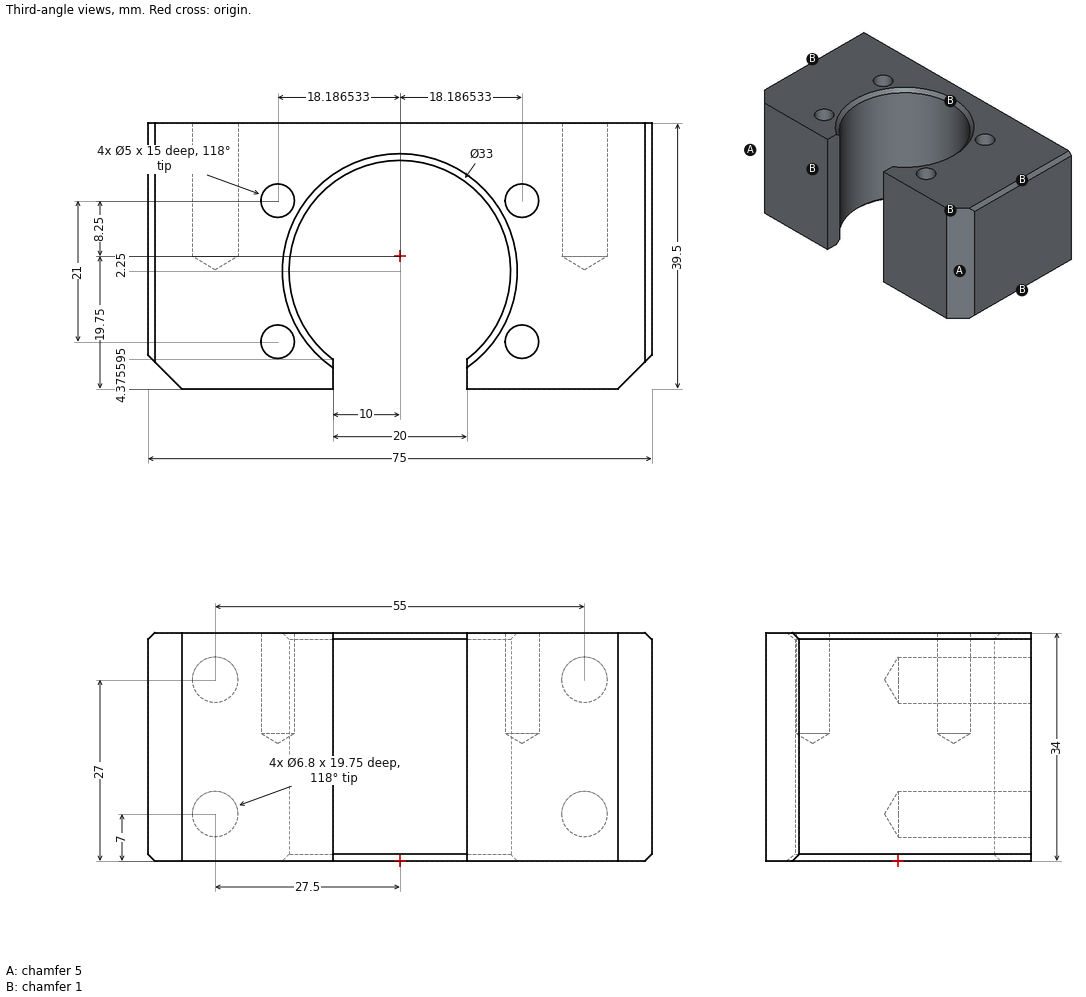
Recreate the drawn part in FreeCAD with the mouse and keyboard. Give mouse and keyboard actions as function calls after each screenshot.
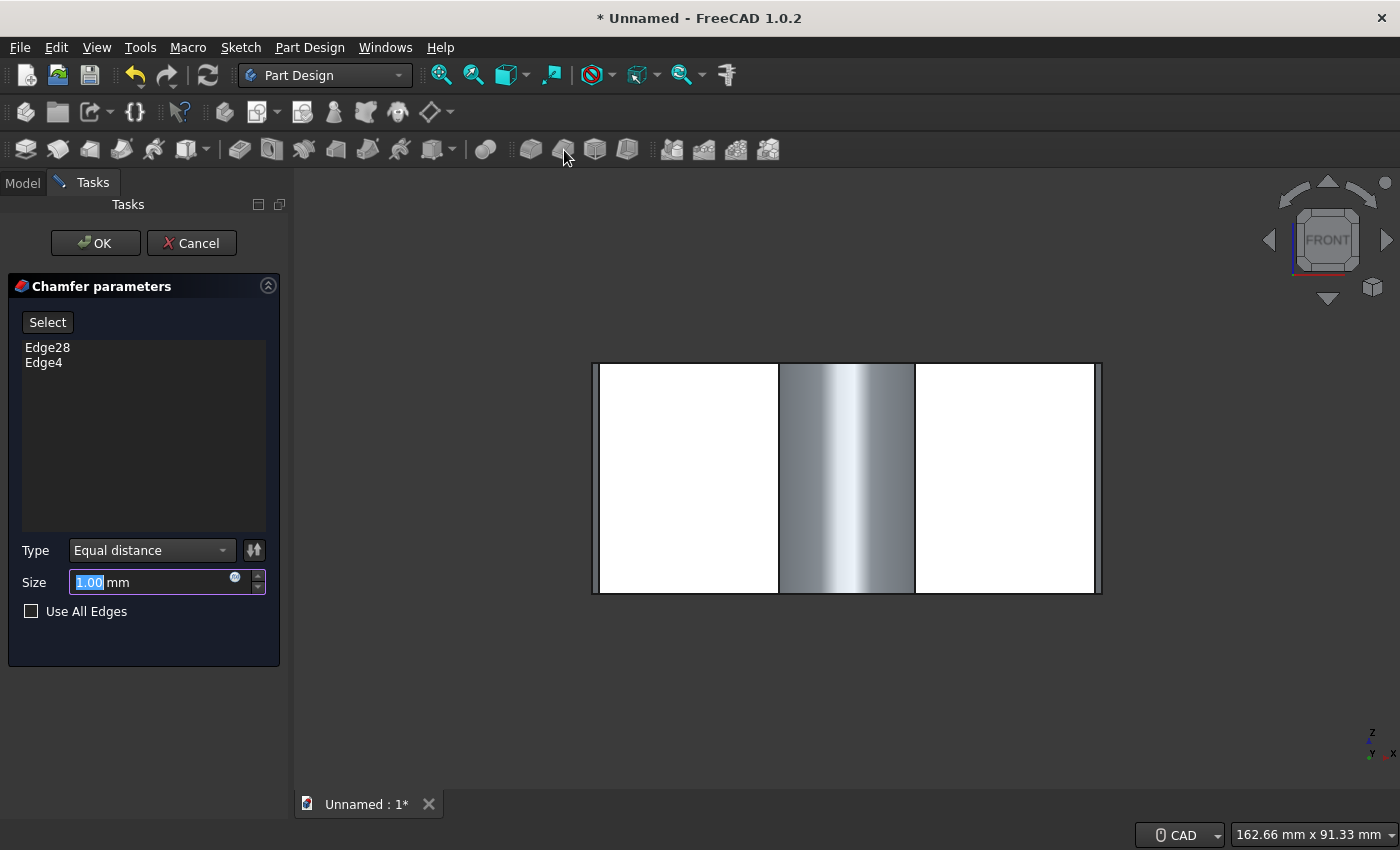
text(5)
key(Tab)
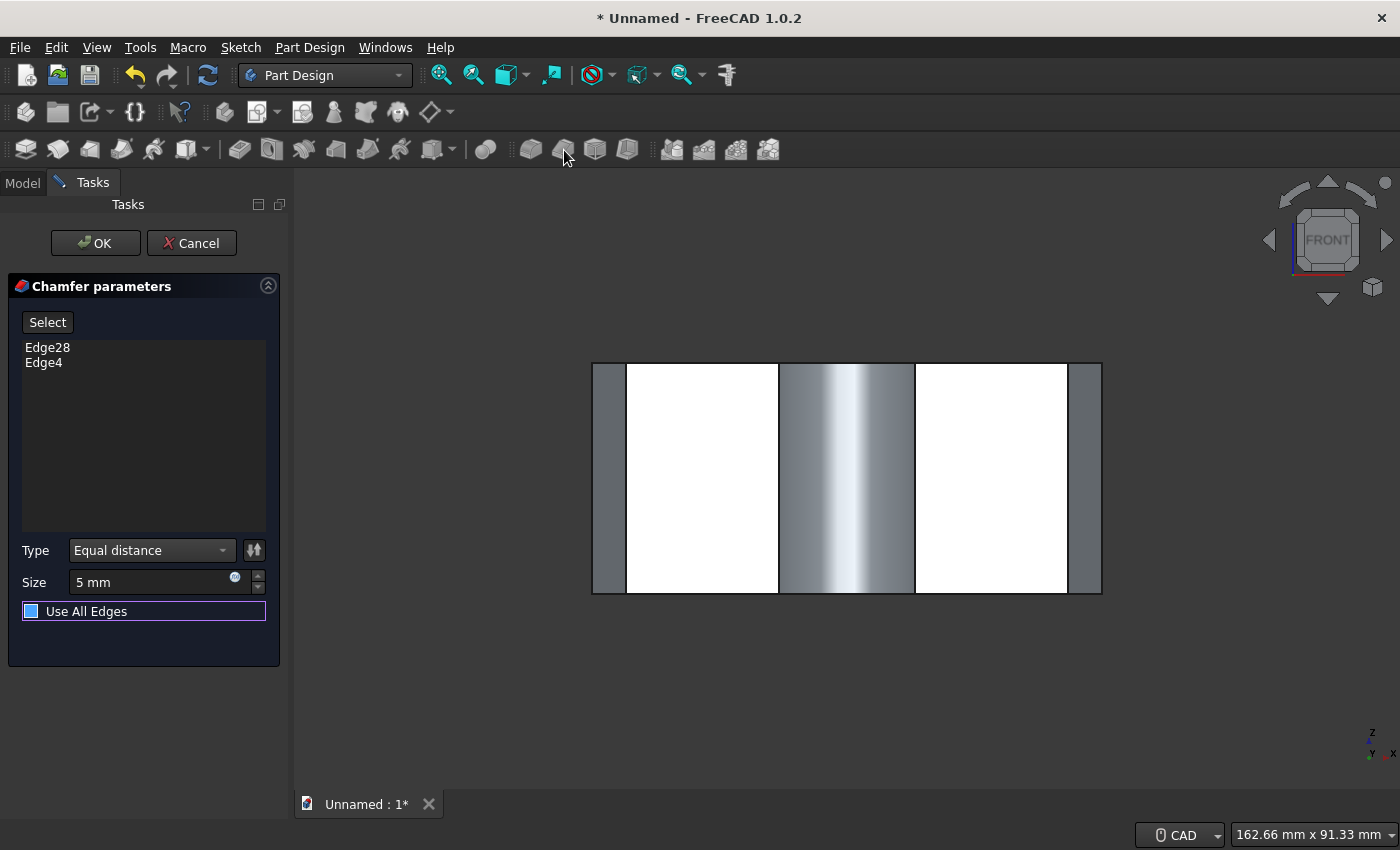
click(96, 243)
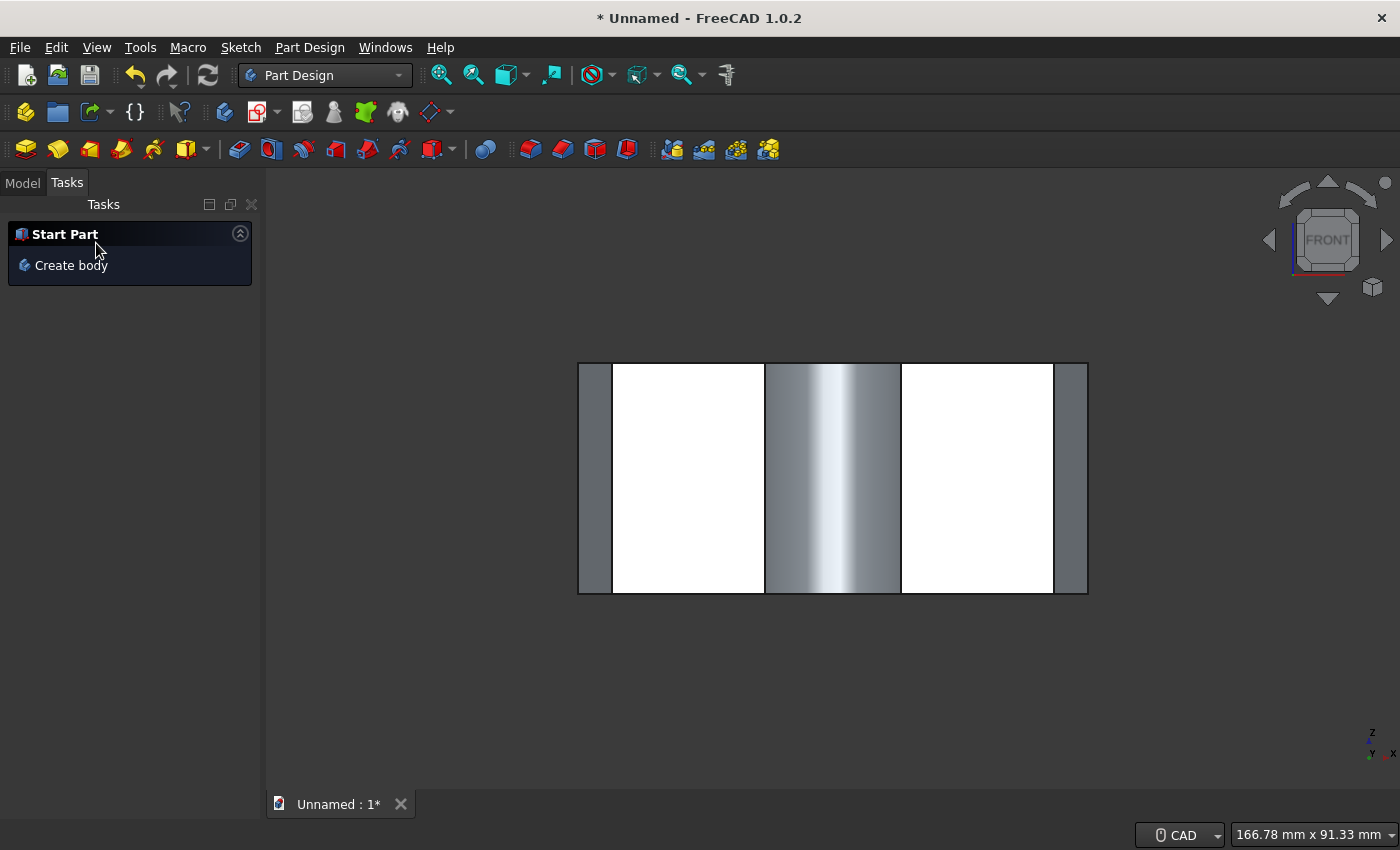
click(442, 76)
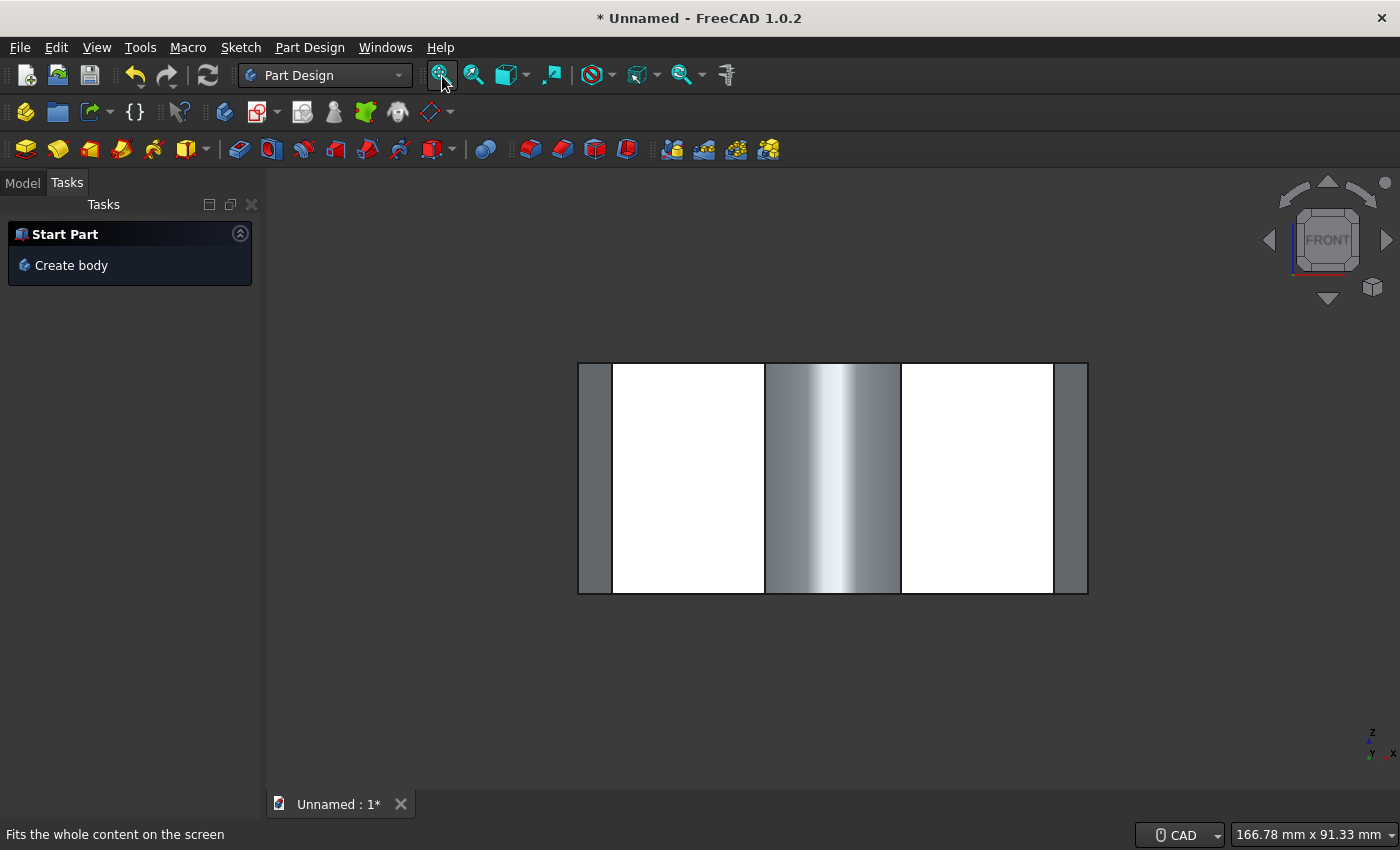
click(783, 593)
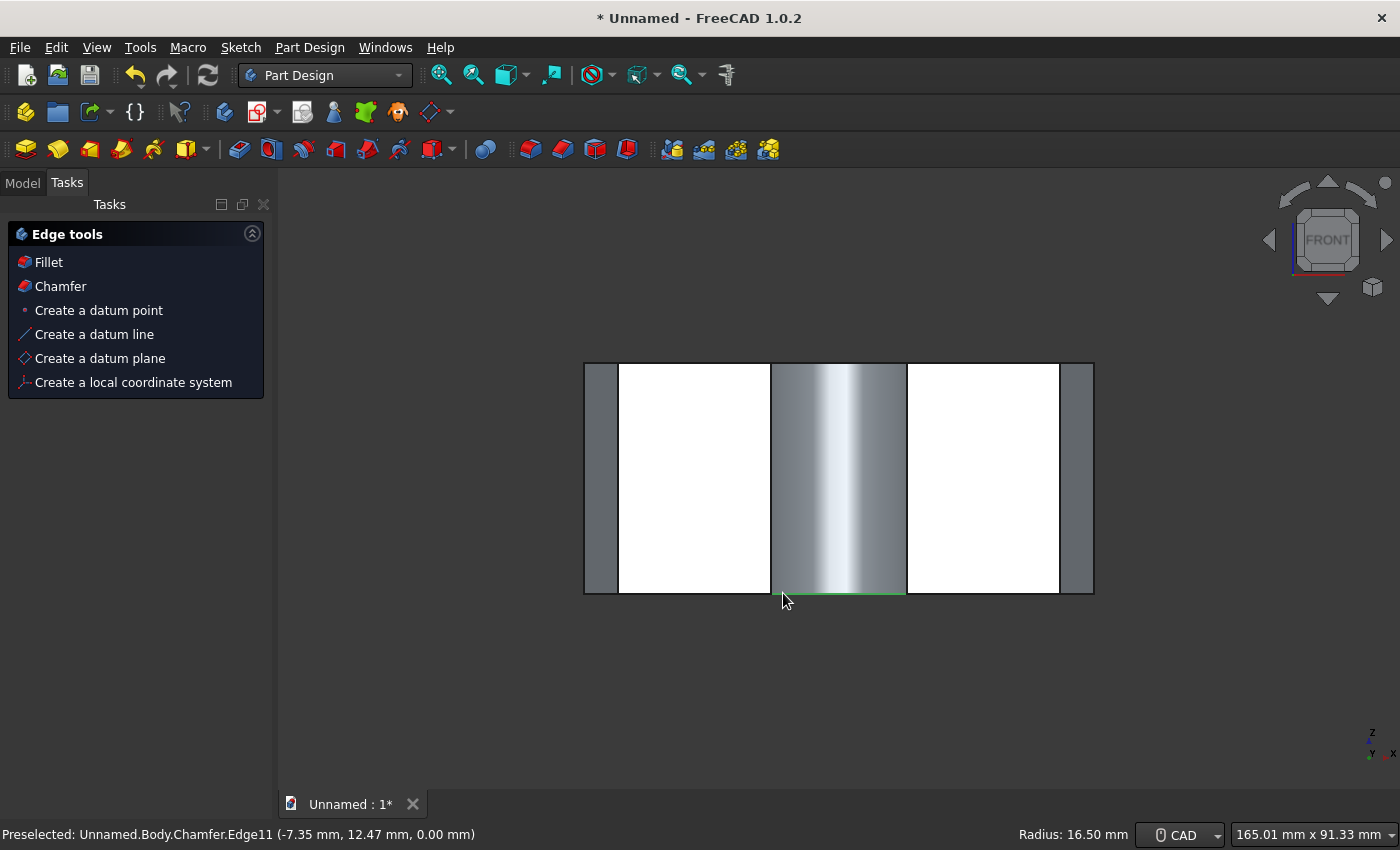
click(789, 362, ctrl)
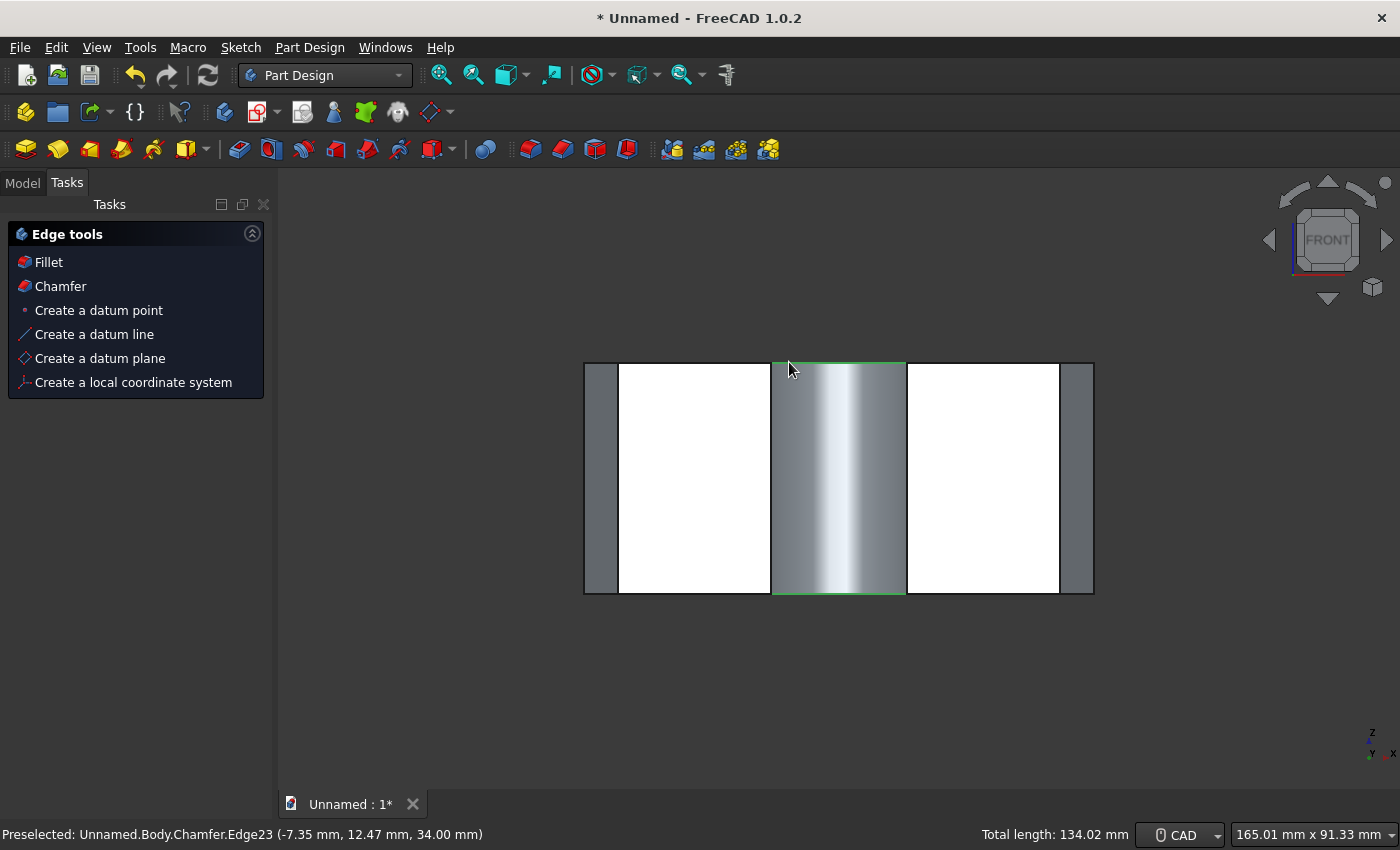
key(0)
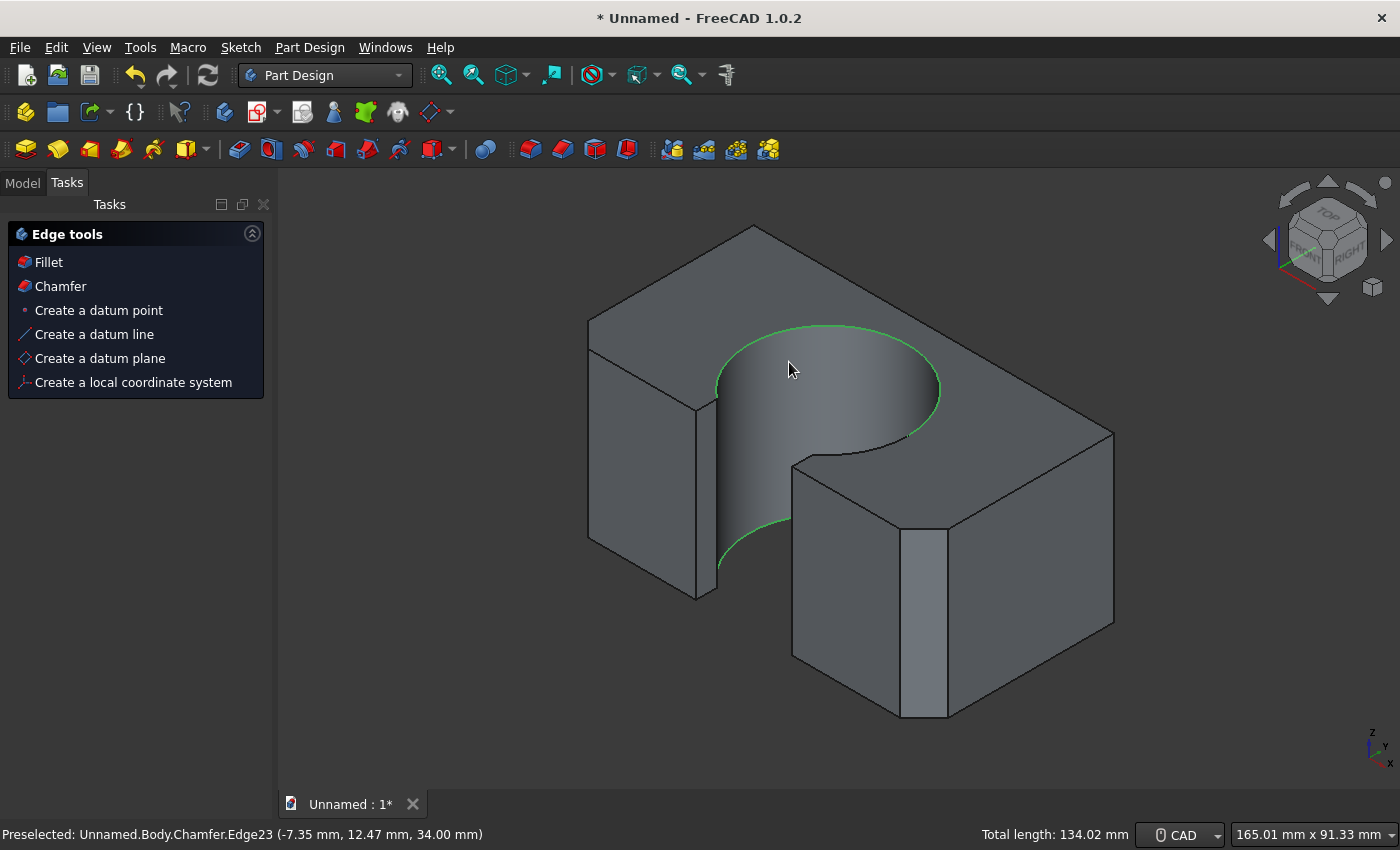
click(1031, 480, ctrl)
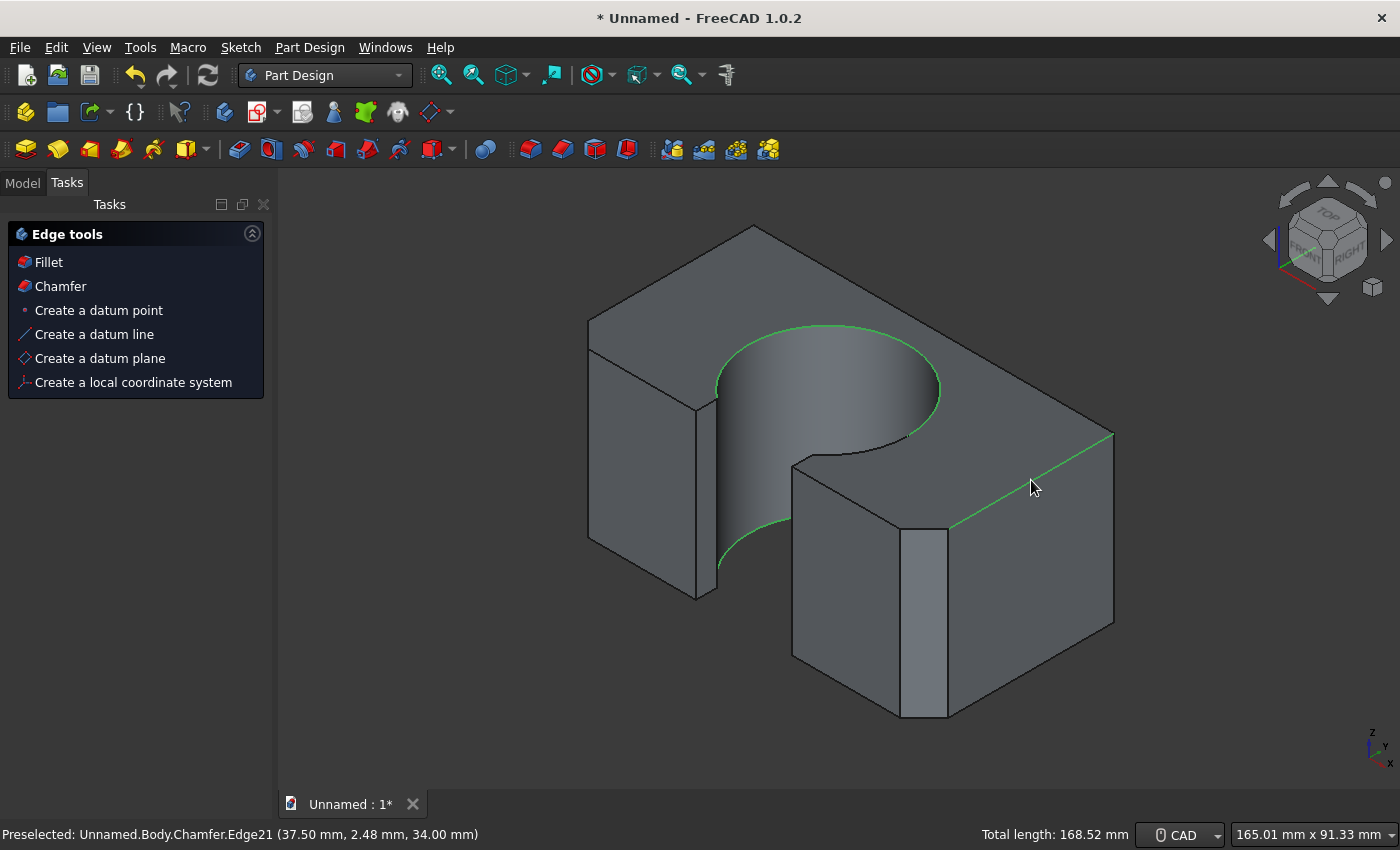
key(2)